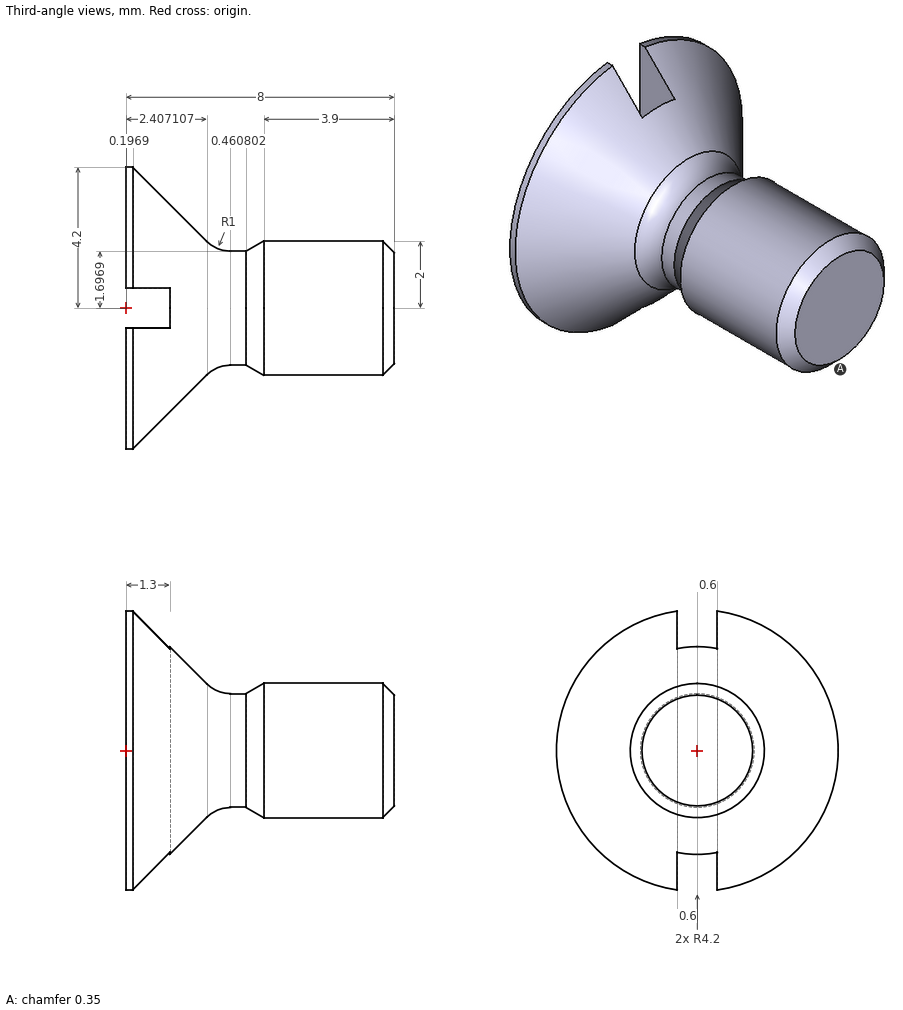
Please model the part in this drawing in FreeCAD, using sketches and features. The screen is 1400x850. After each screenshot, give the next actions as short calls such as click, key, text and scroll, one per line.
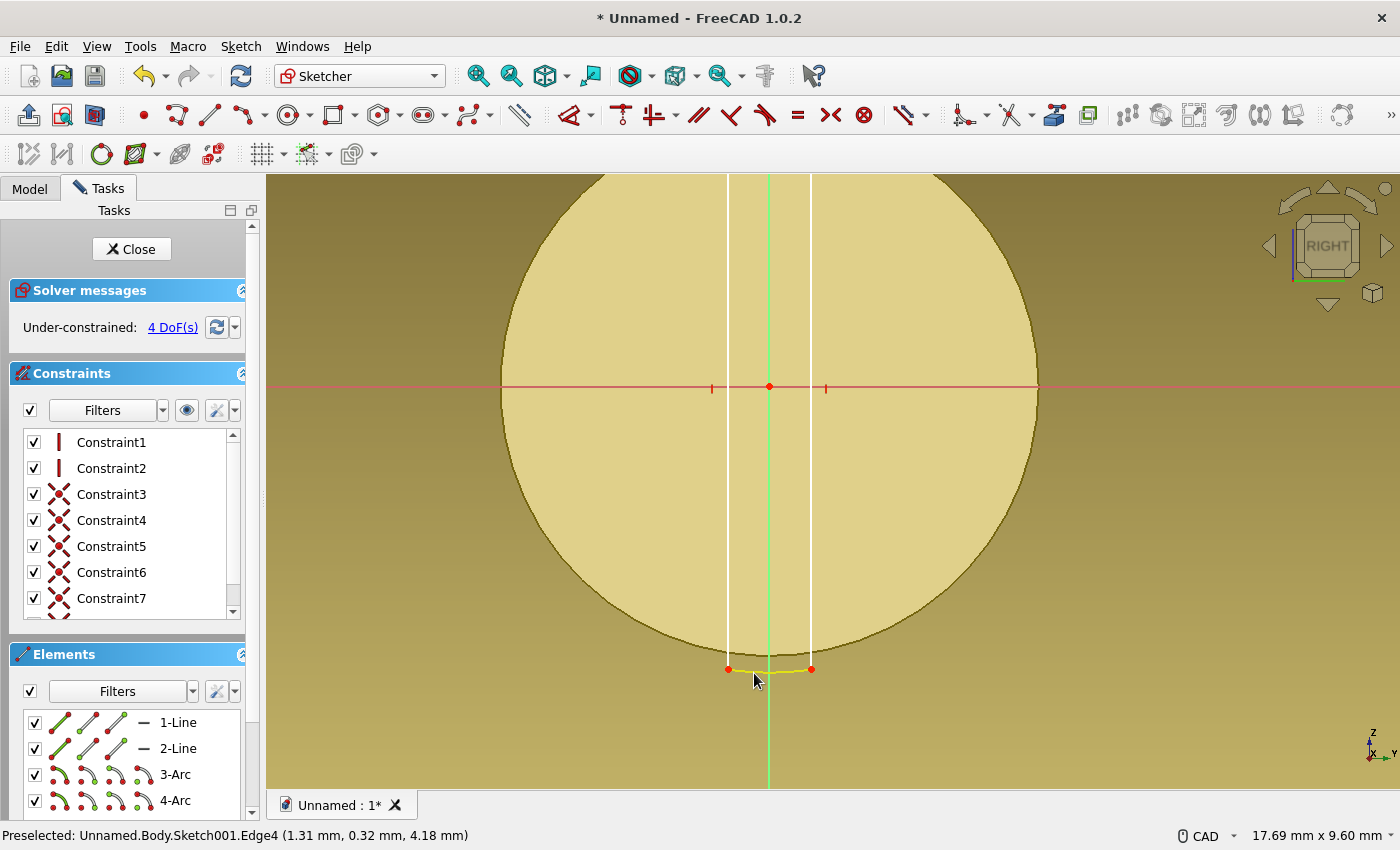
click(753, 672)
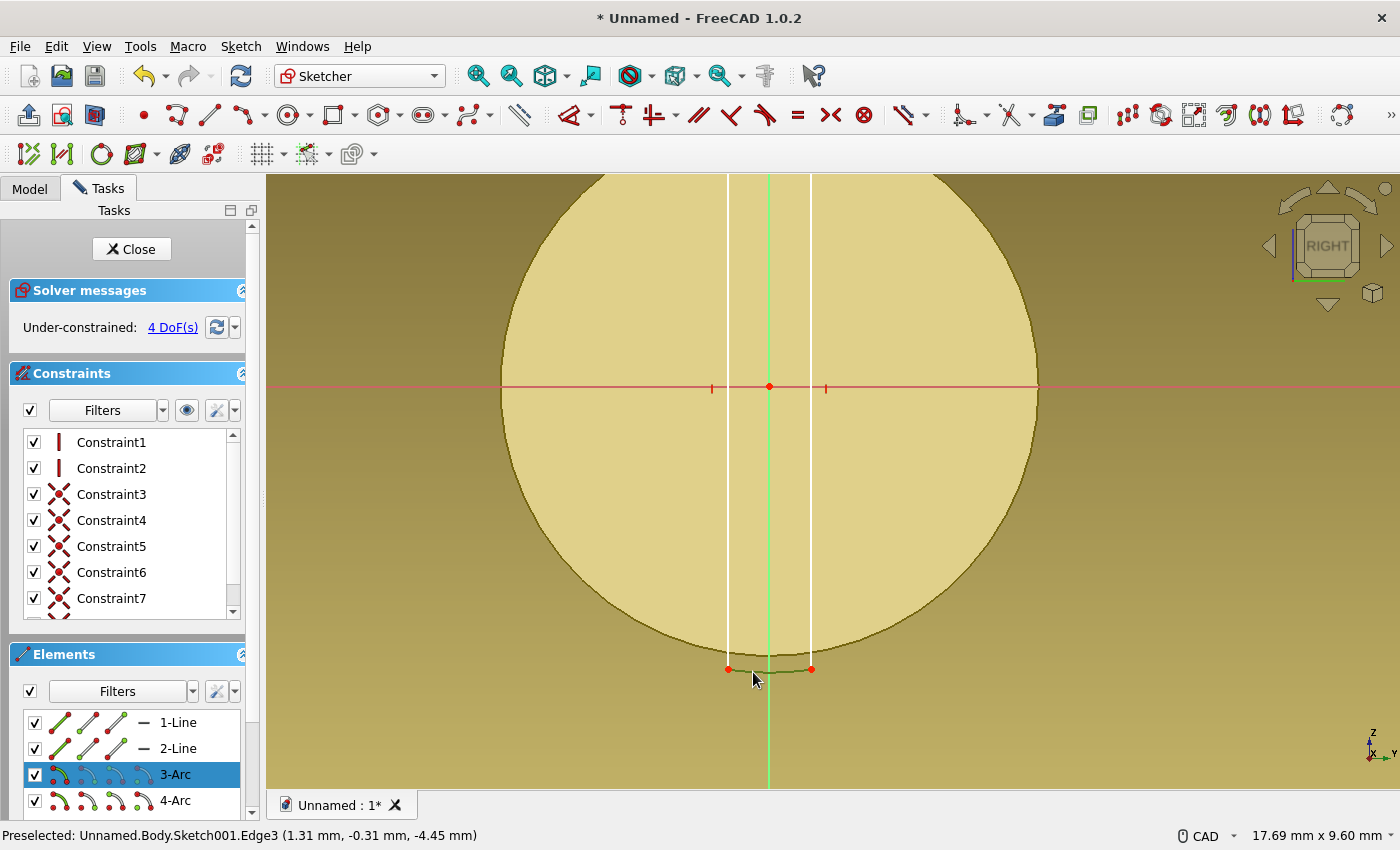
scroll(754, 674, down, 2)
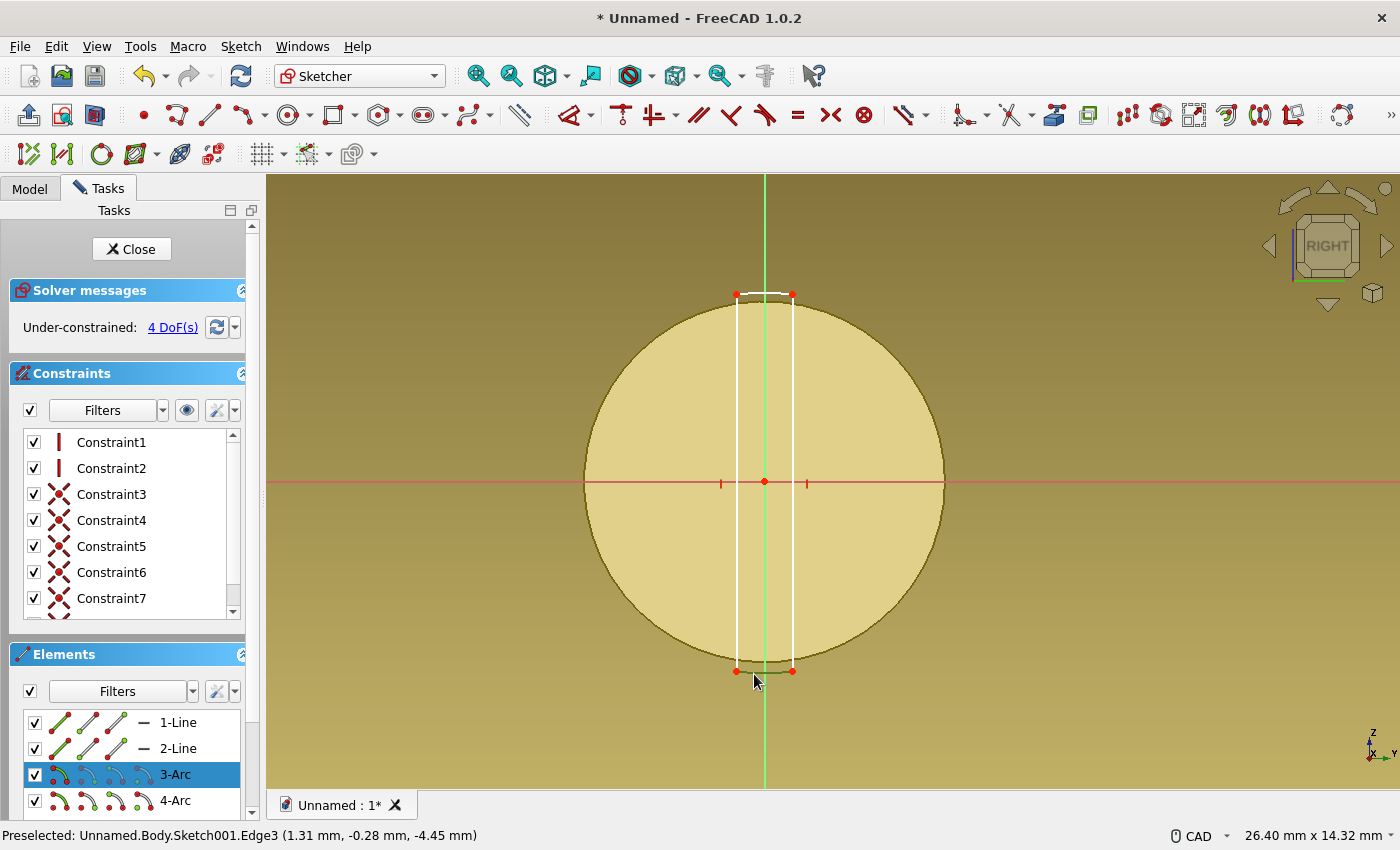
click(776, 293)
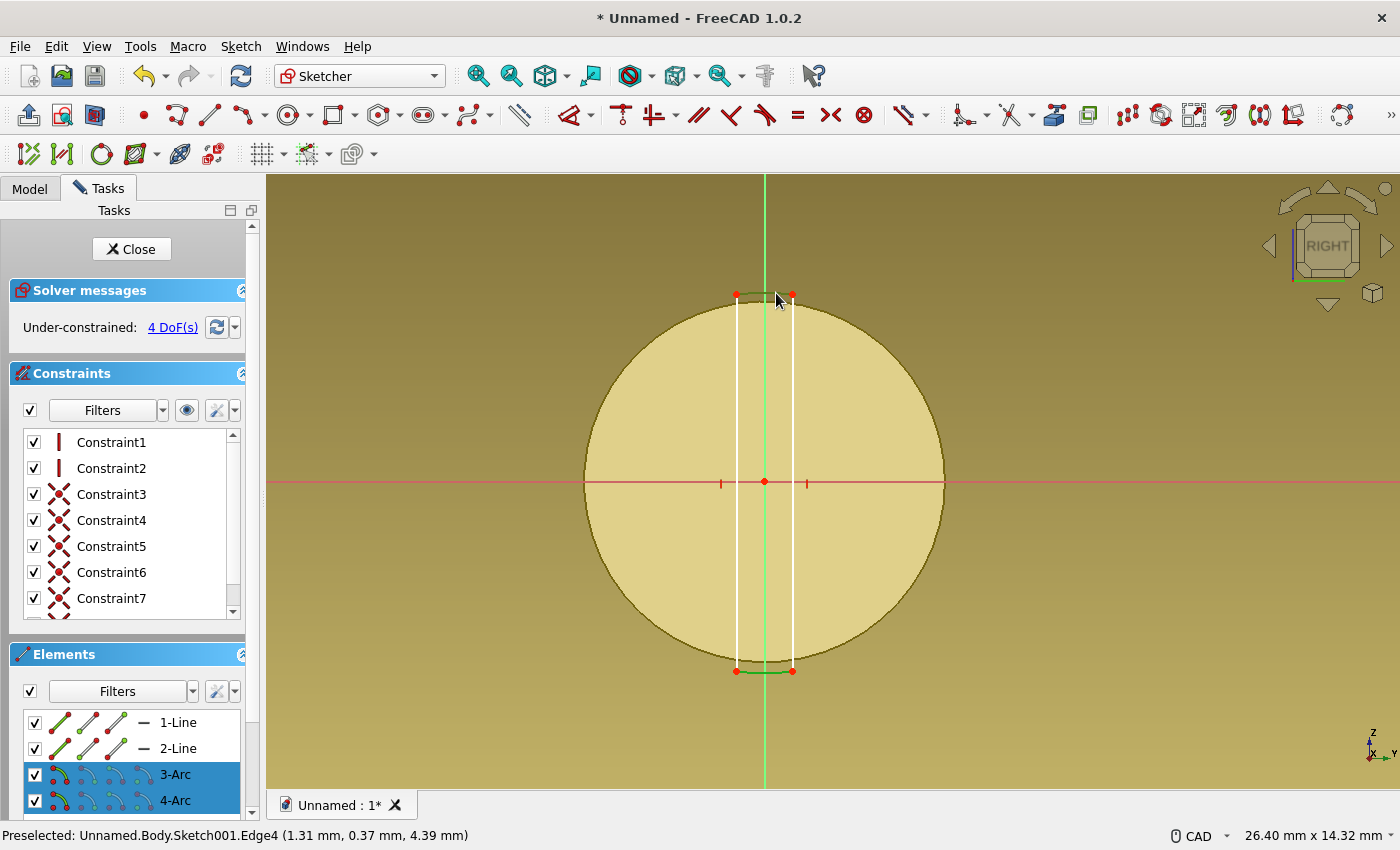
key(e)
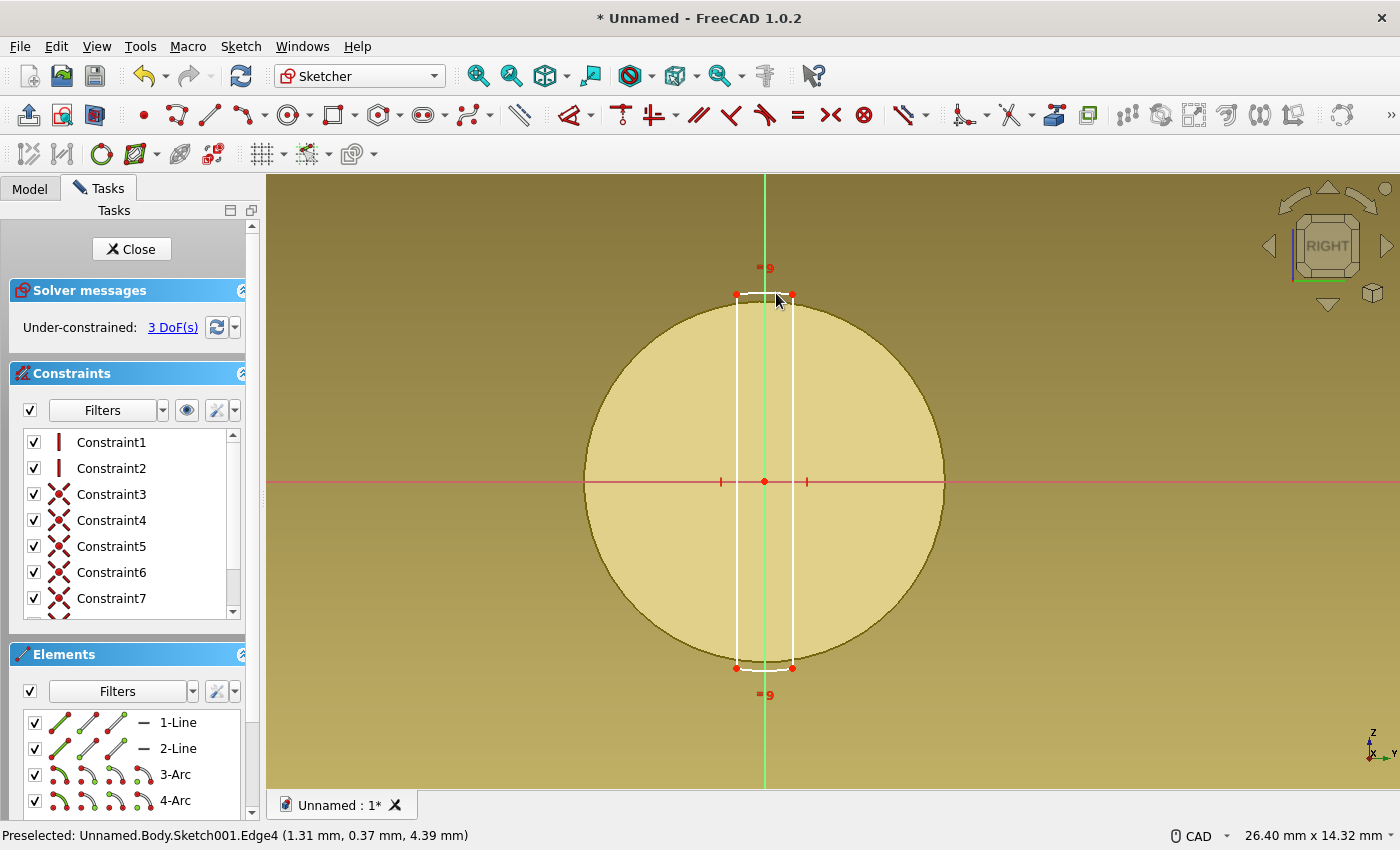
key(d)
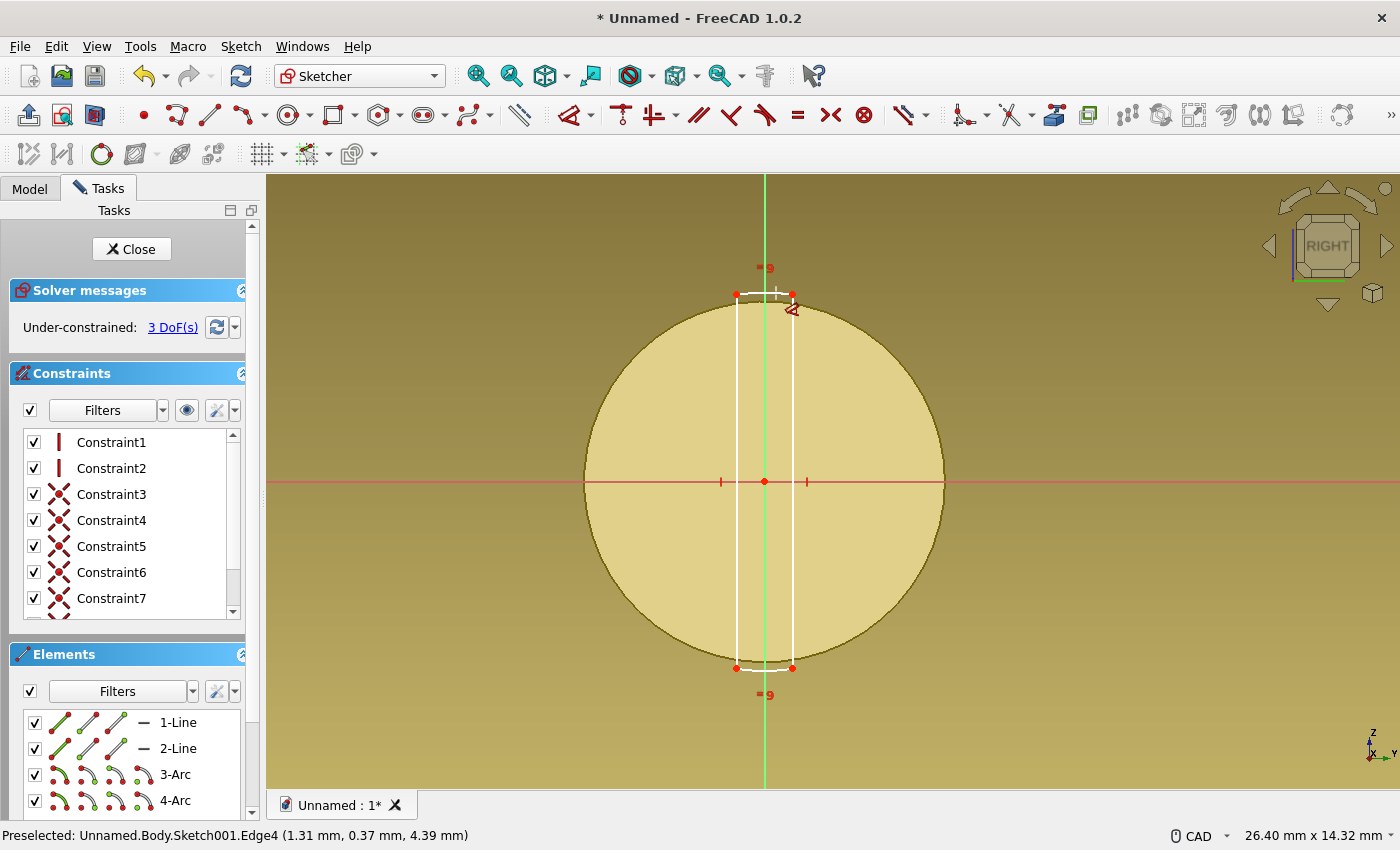
scroll(754, 671, up, 2)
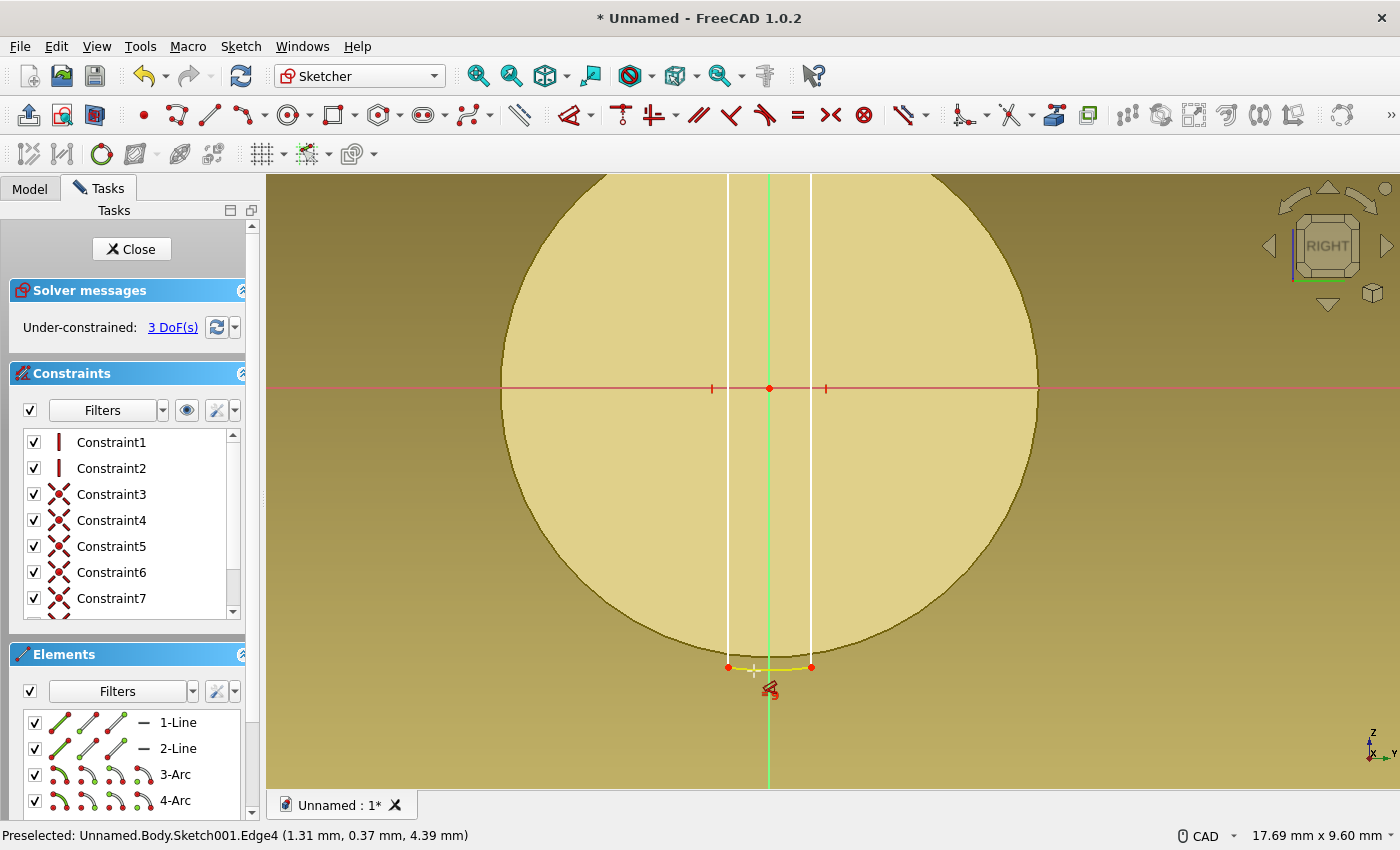
click(753, 670)
click(751, 702)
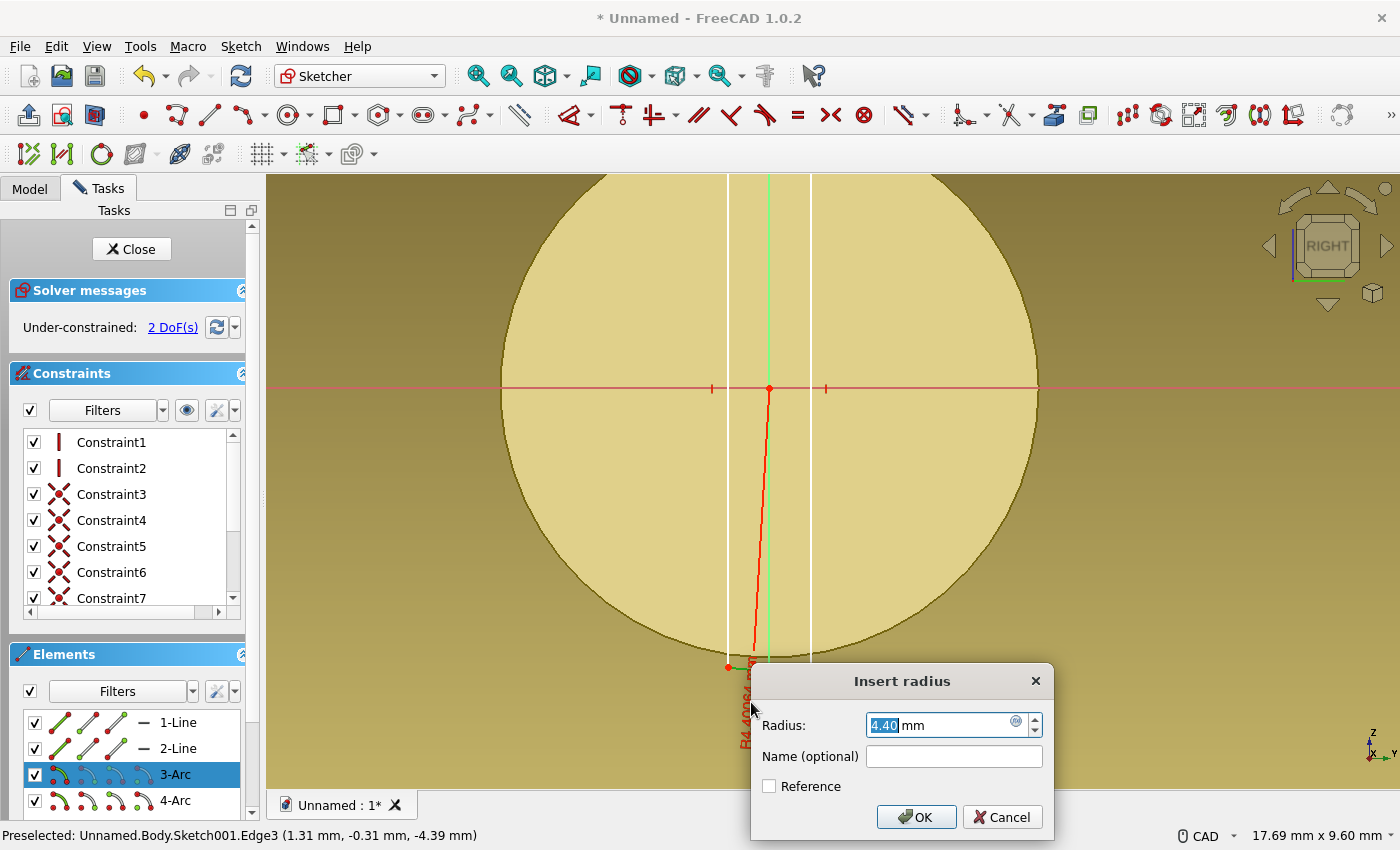
text(4.2)
key(Return)